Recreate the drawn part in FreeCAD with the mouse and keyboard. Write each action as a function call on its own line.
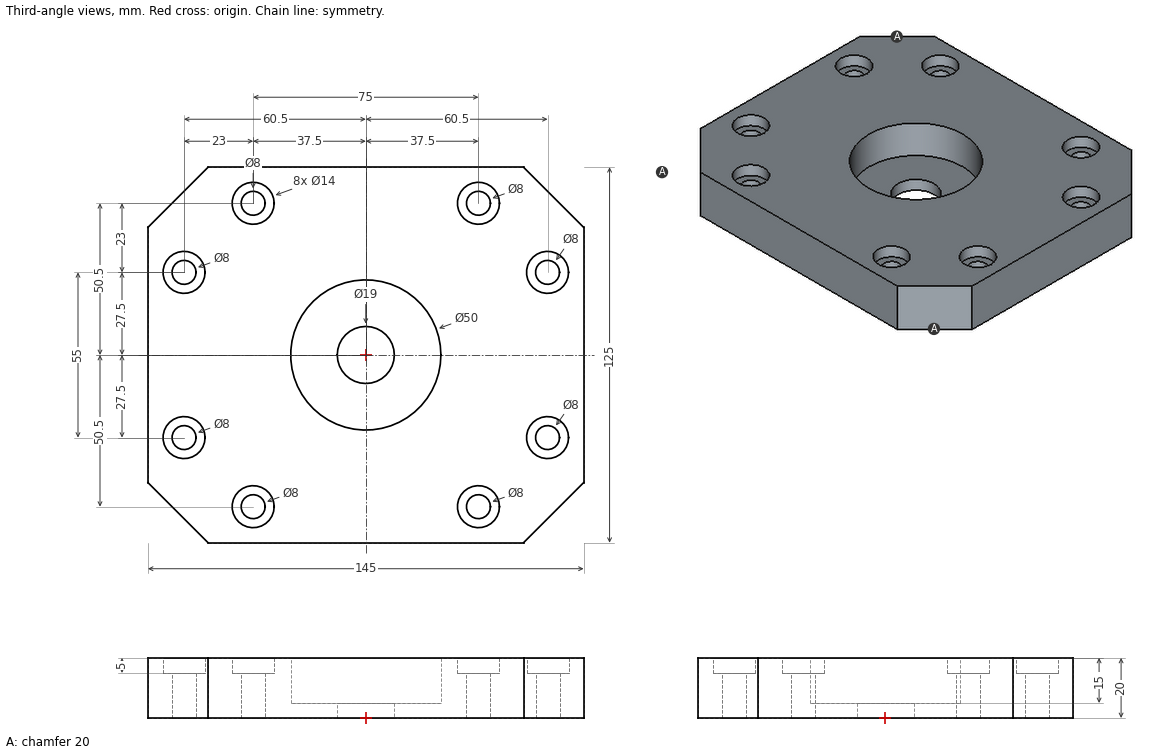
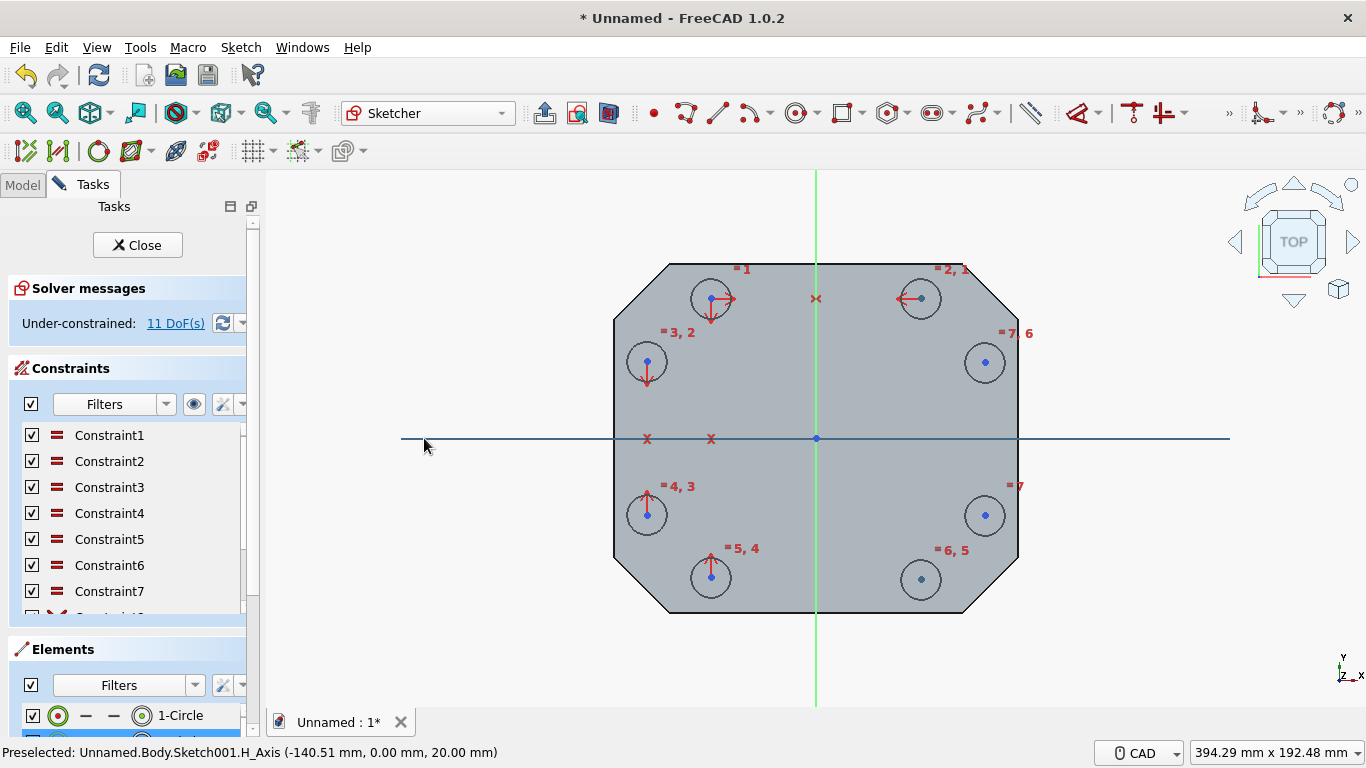
key(s)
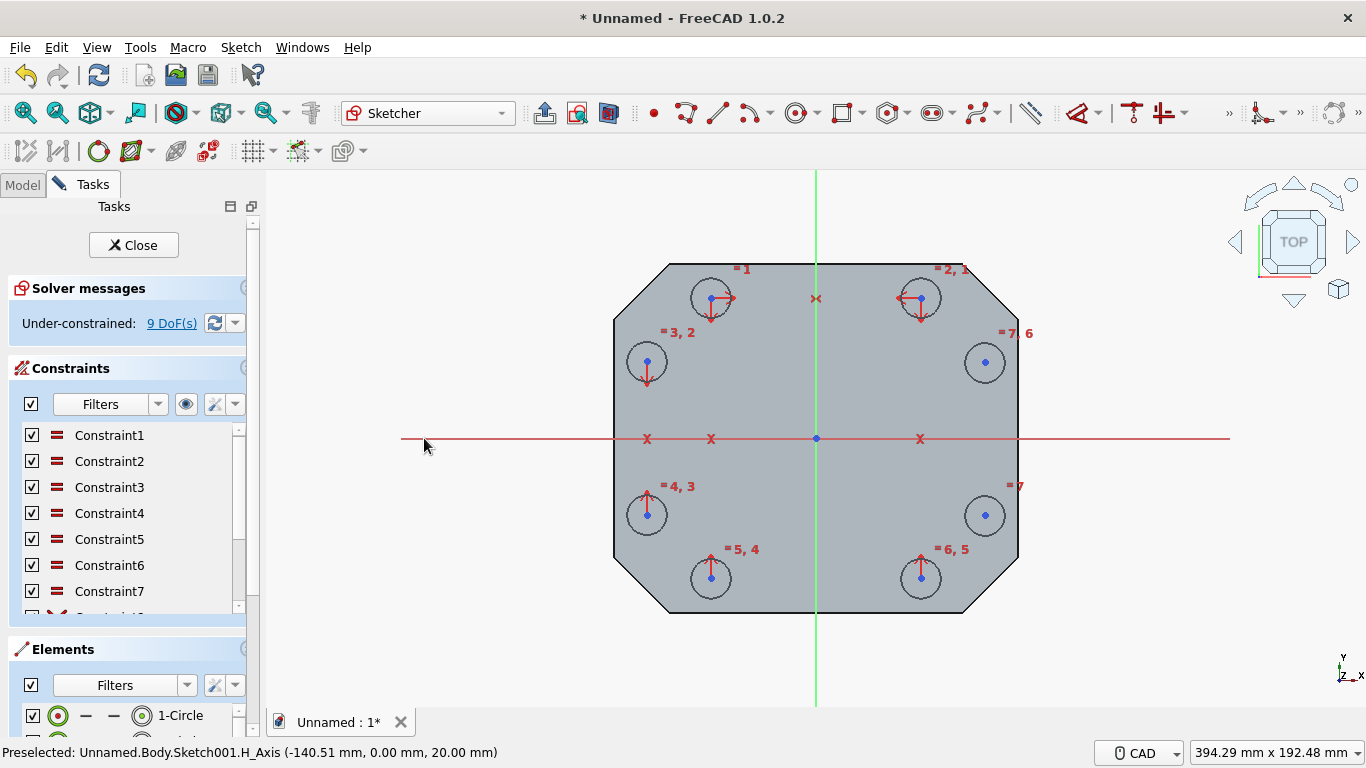
click(647, 362)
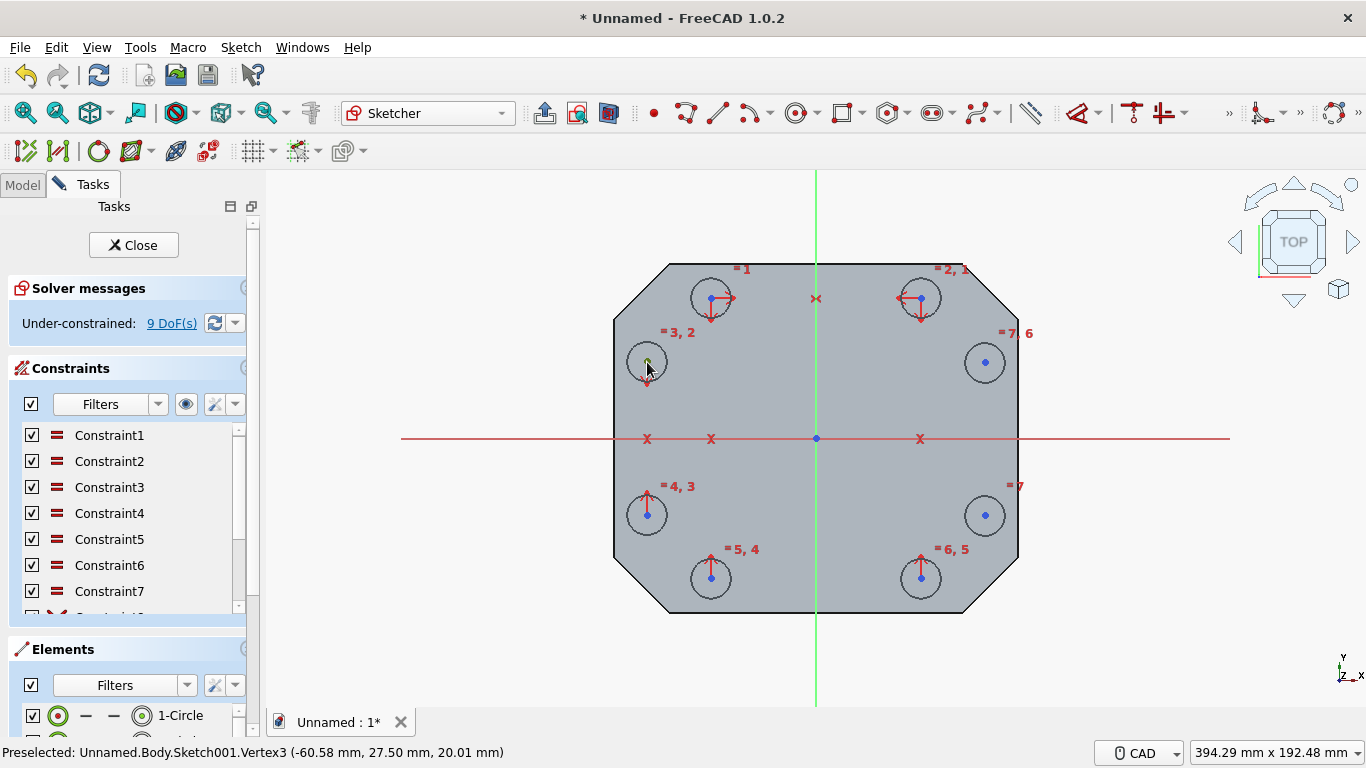
click(985, 363)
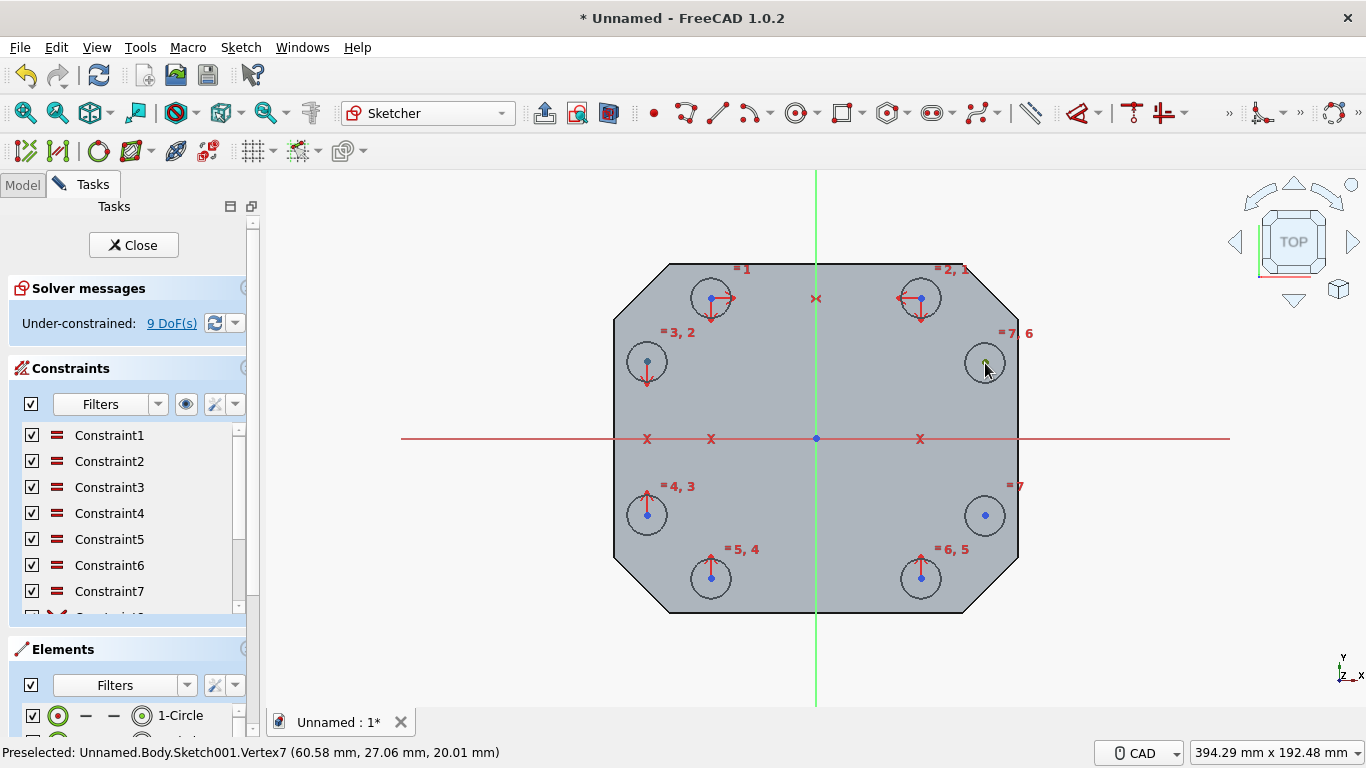
click(816, 645)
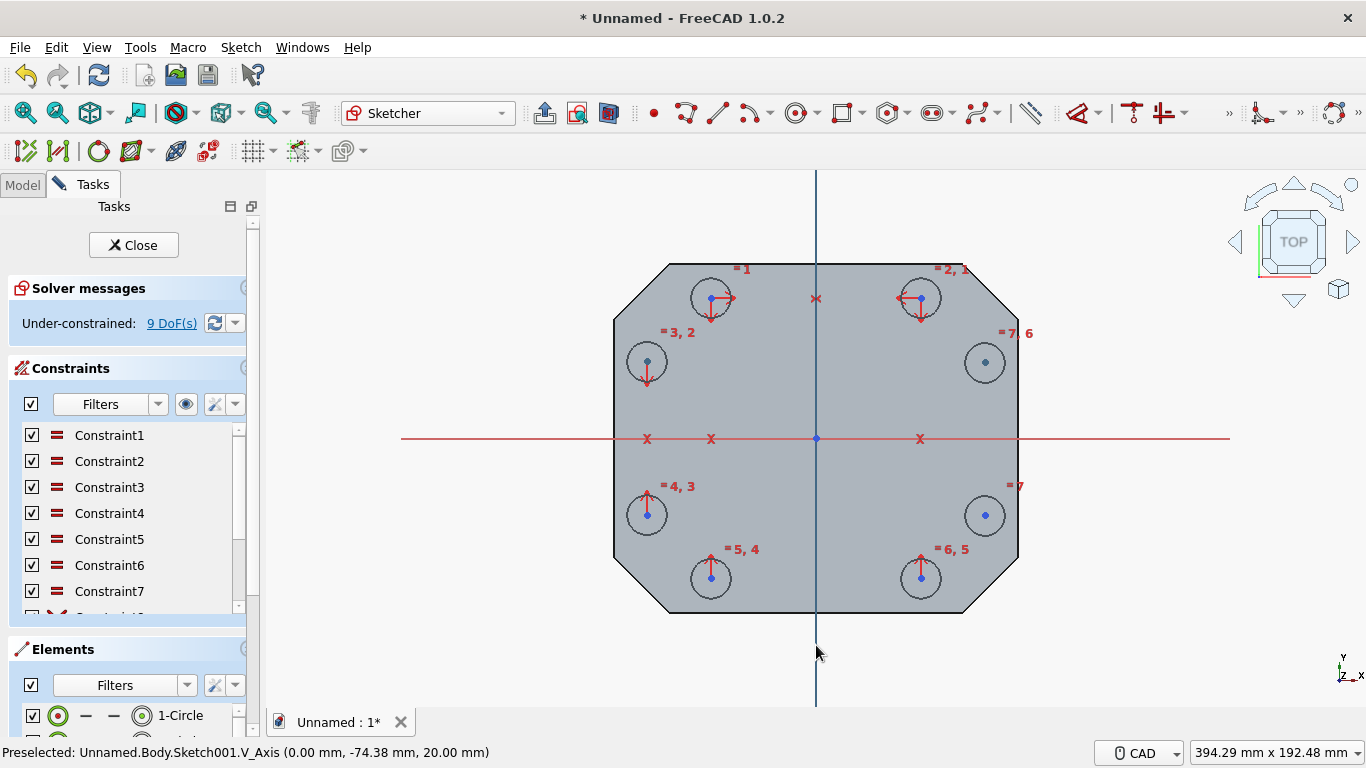
key(s)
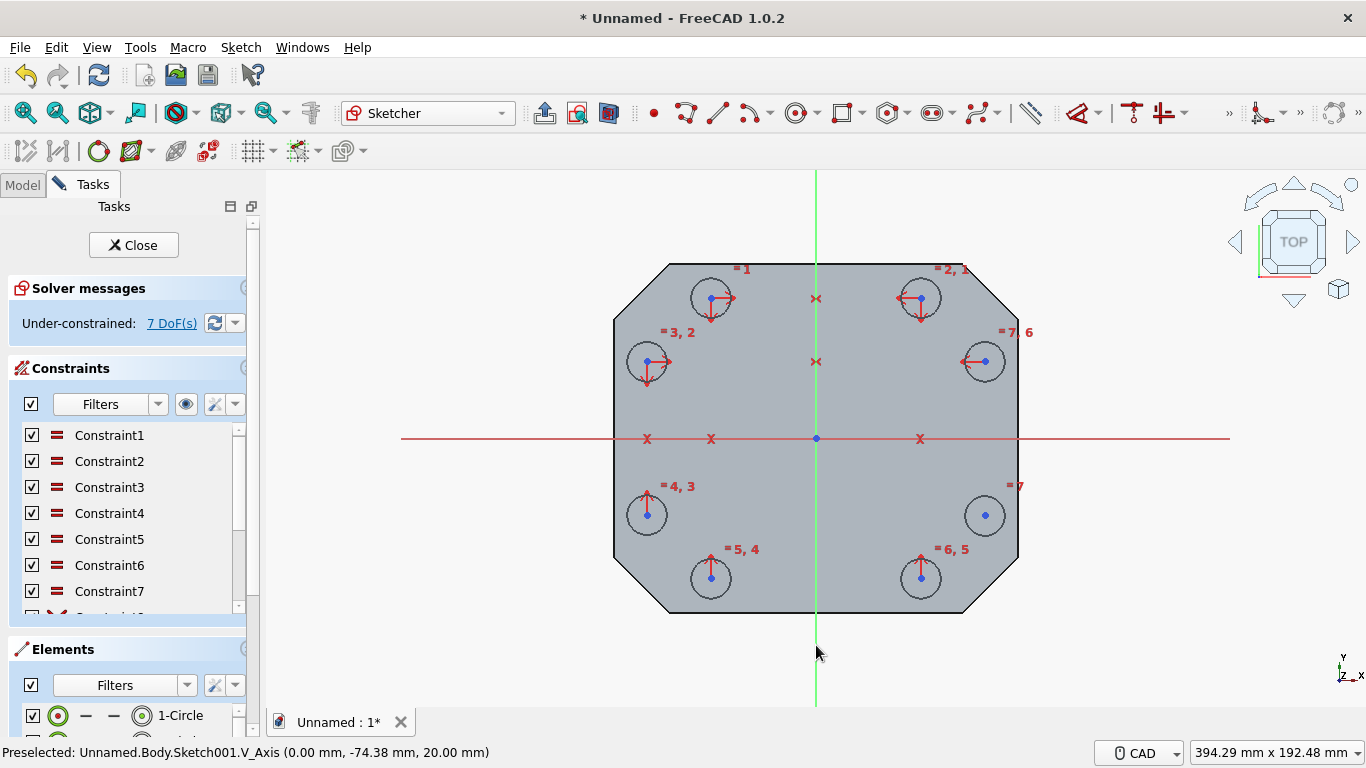
click(647, 515)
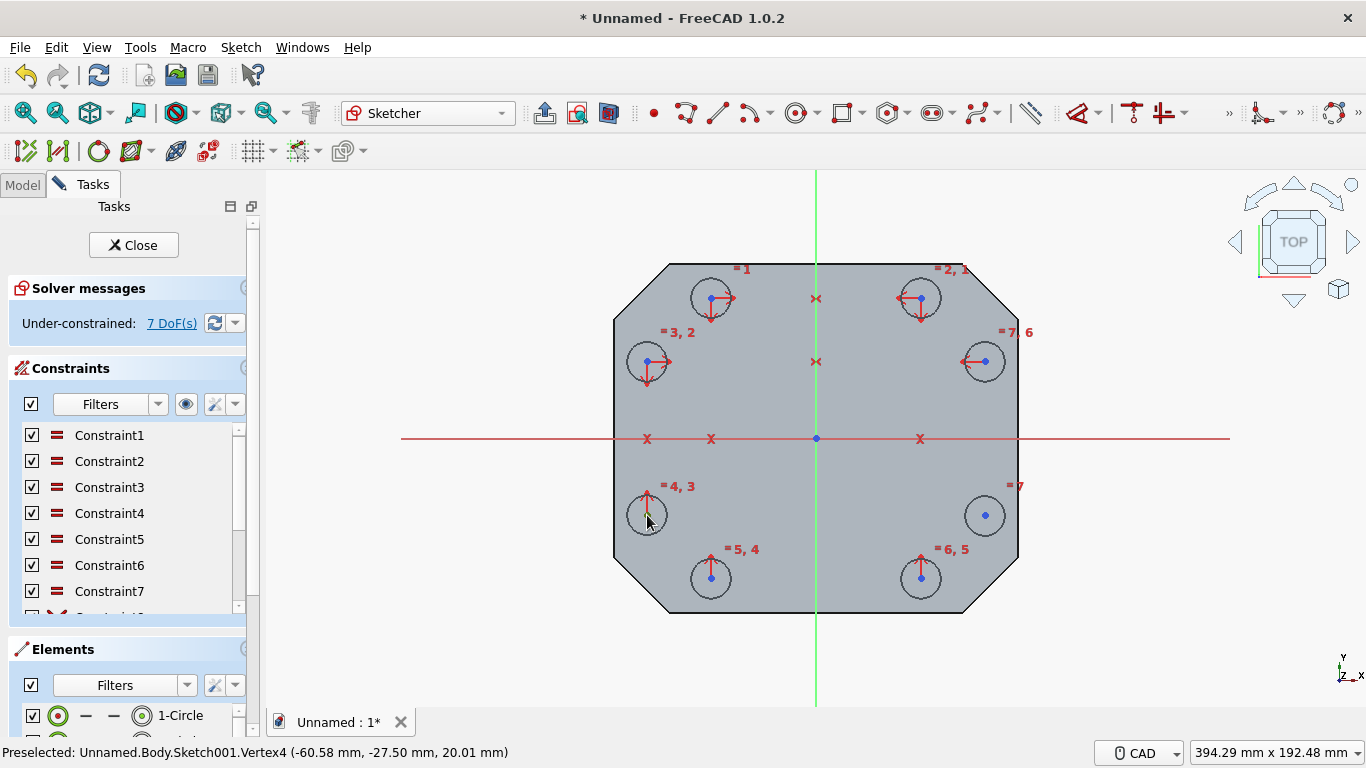
click(985, 516)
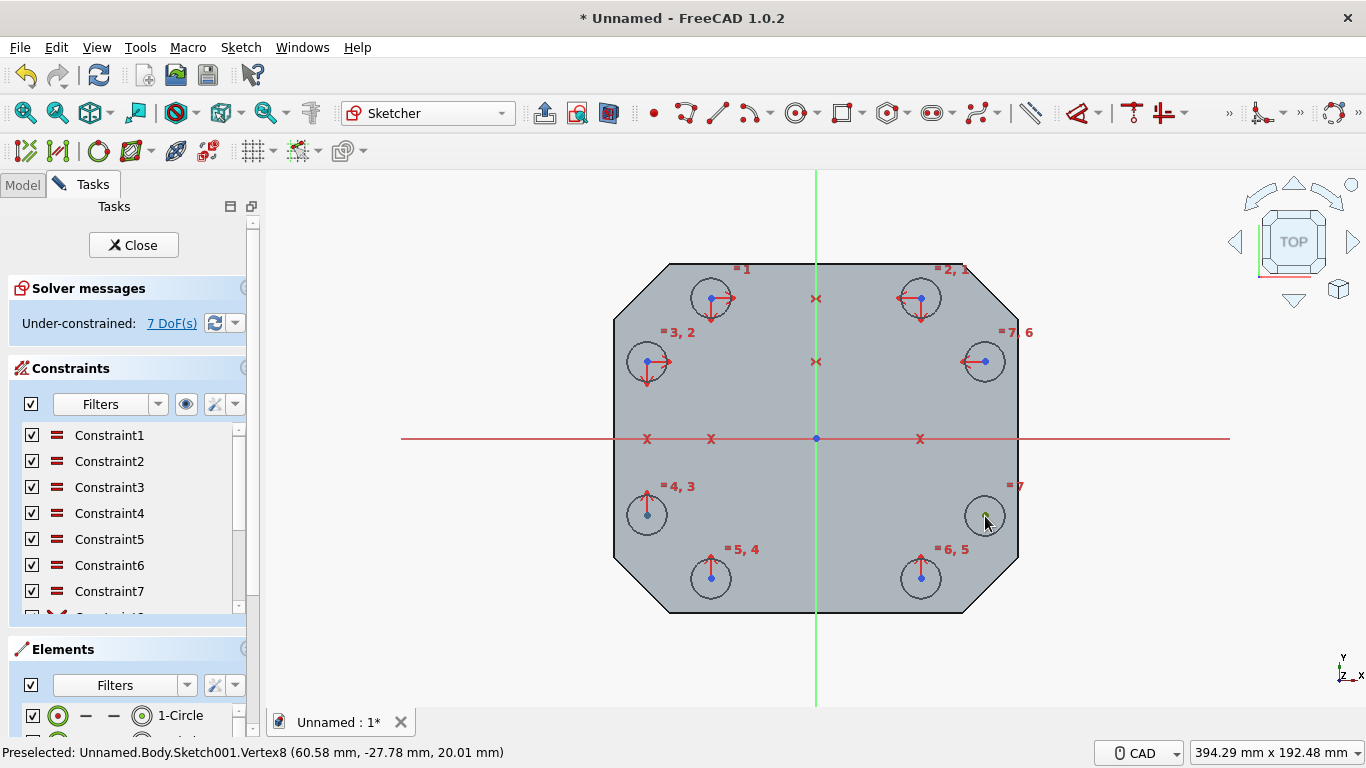
click(816, 645)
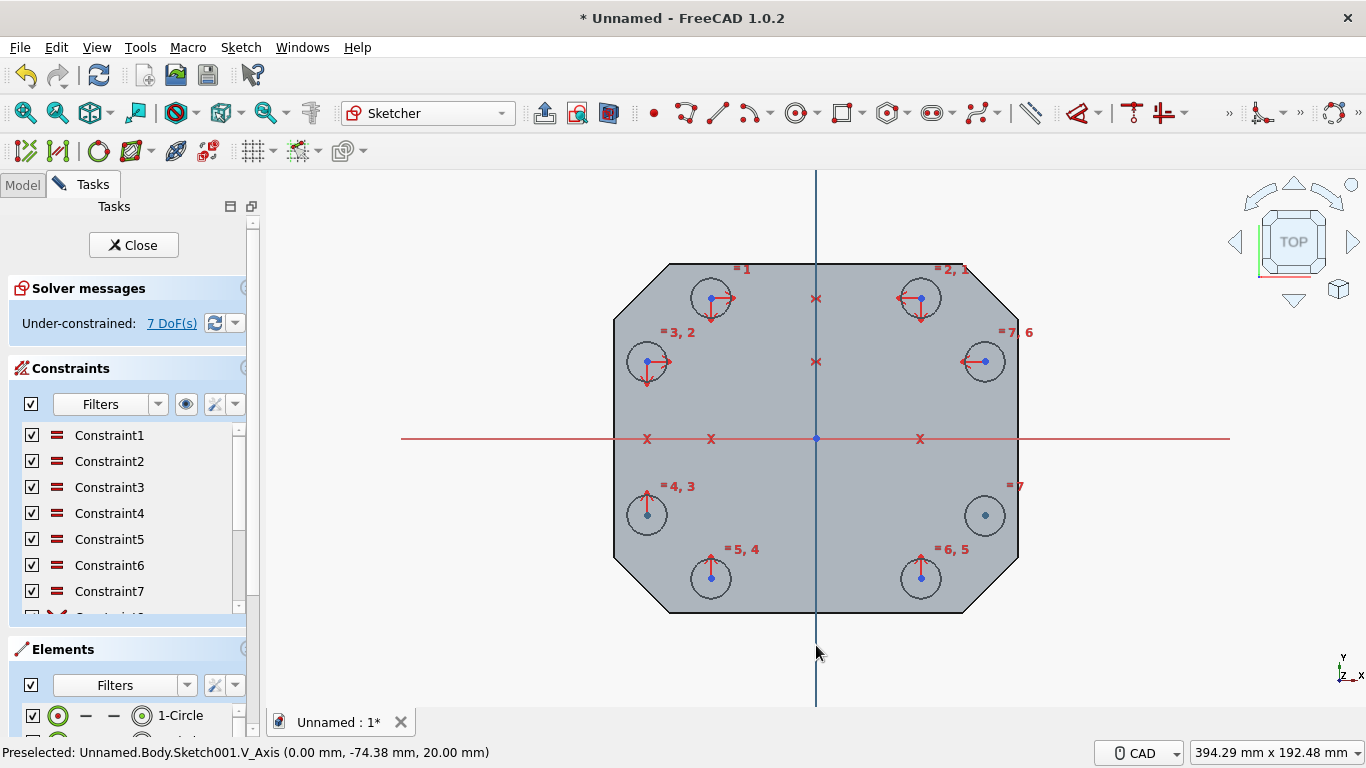
key(s)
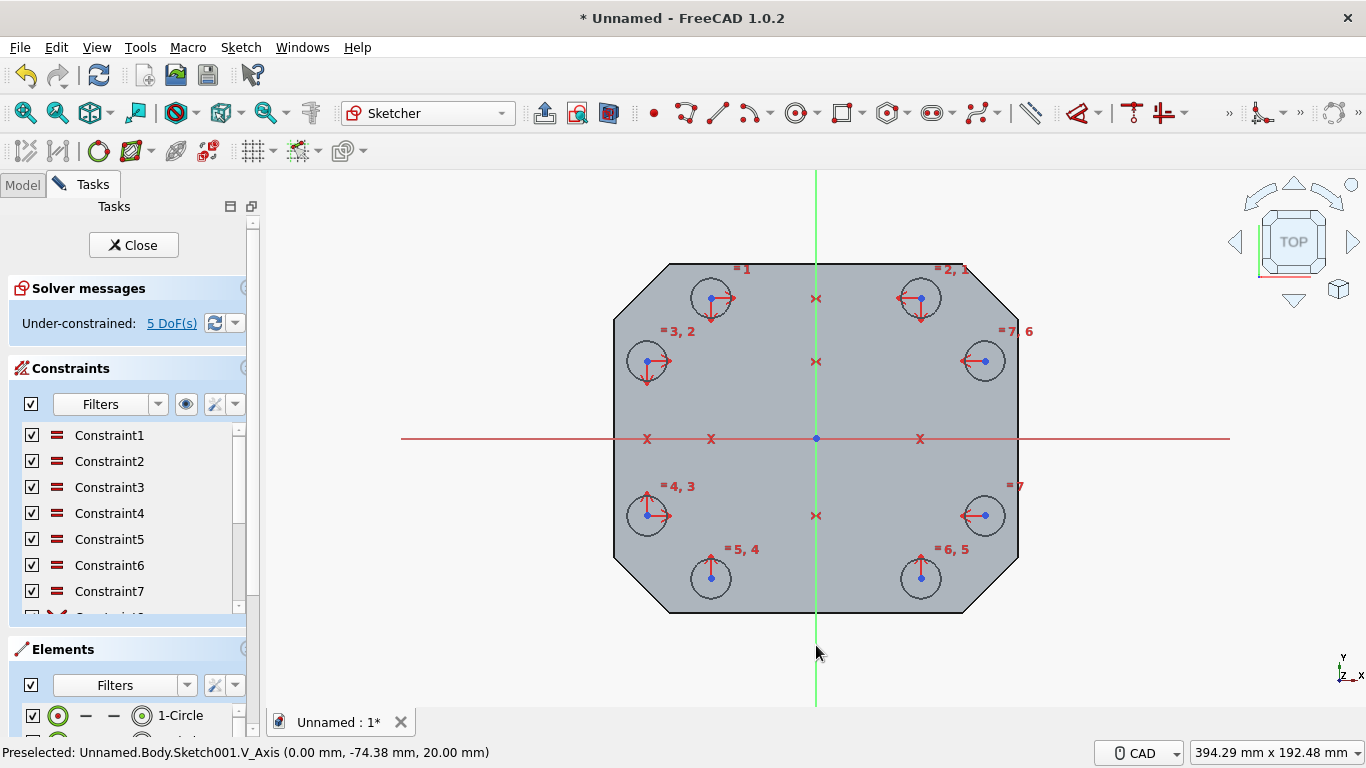
click(1078, 114)